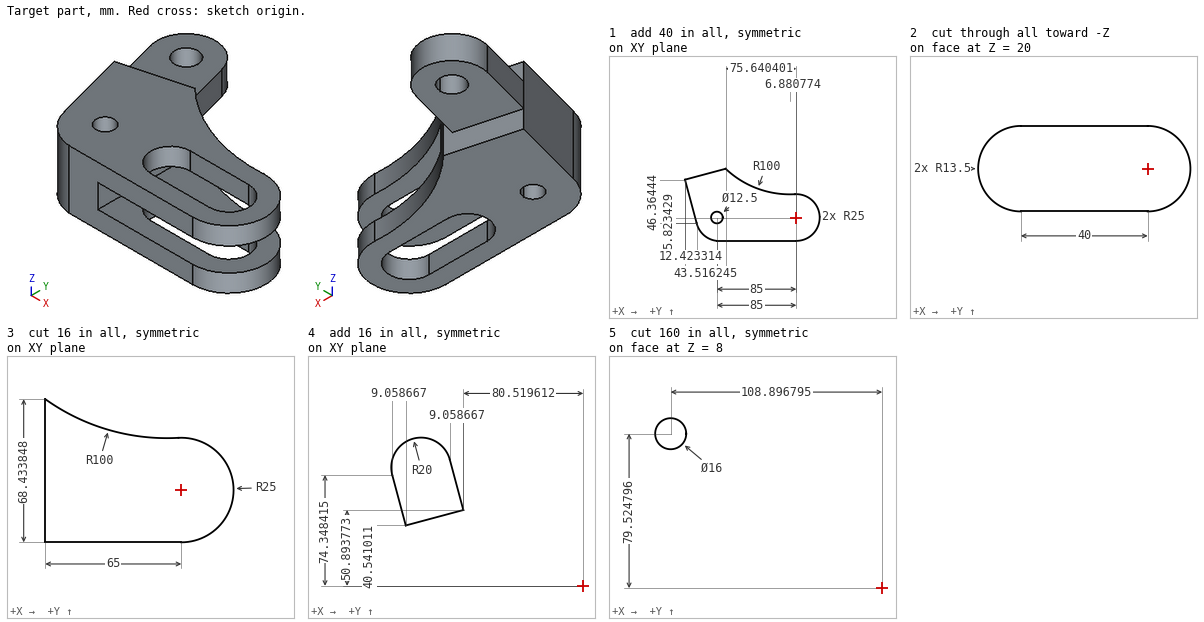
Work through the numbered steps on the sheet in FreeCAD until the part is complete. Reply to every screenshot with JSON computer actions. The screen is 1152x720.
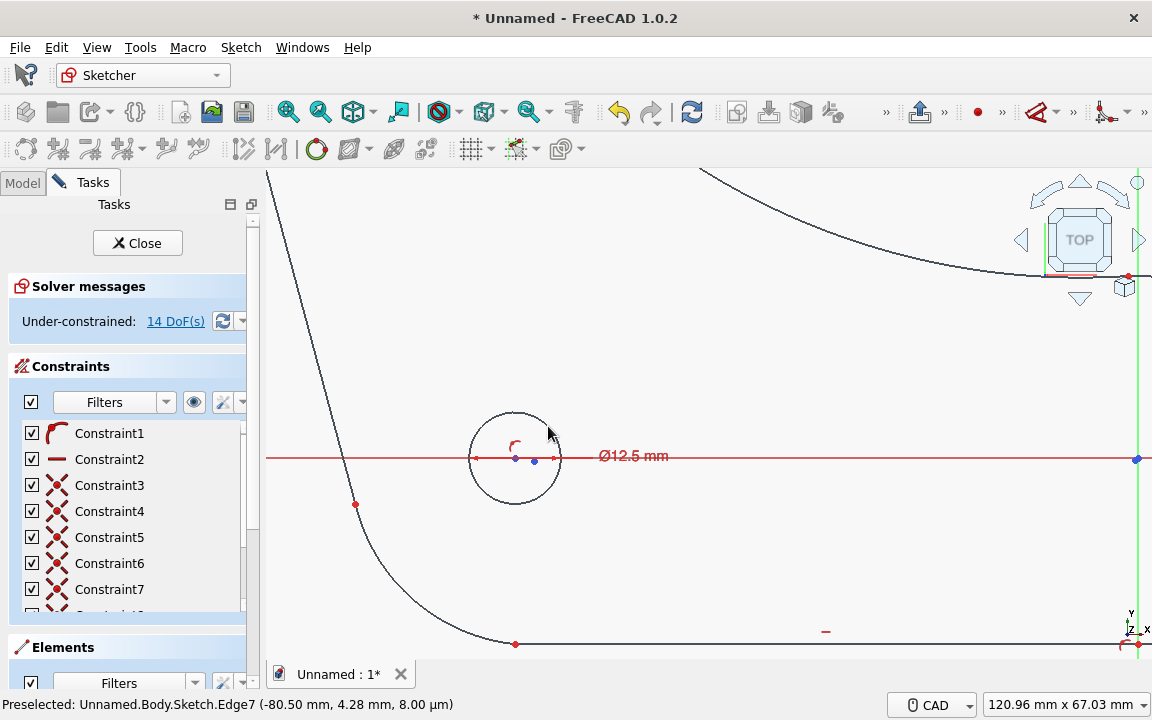
{"action": "scroll", "coordinate": [516, 458], "scroll_direction": "down", "scroll_amount": 4}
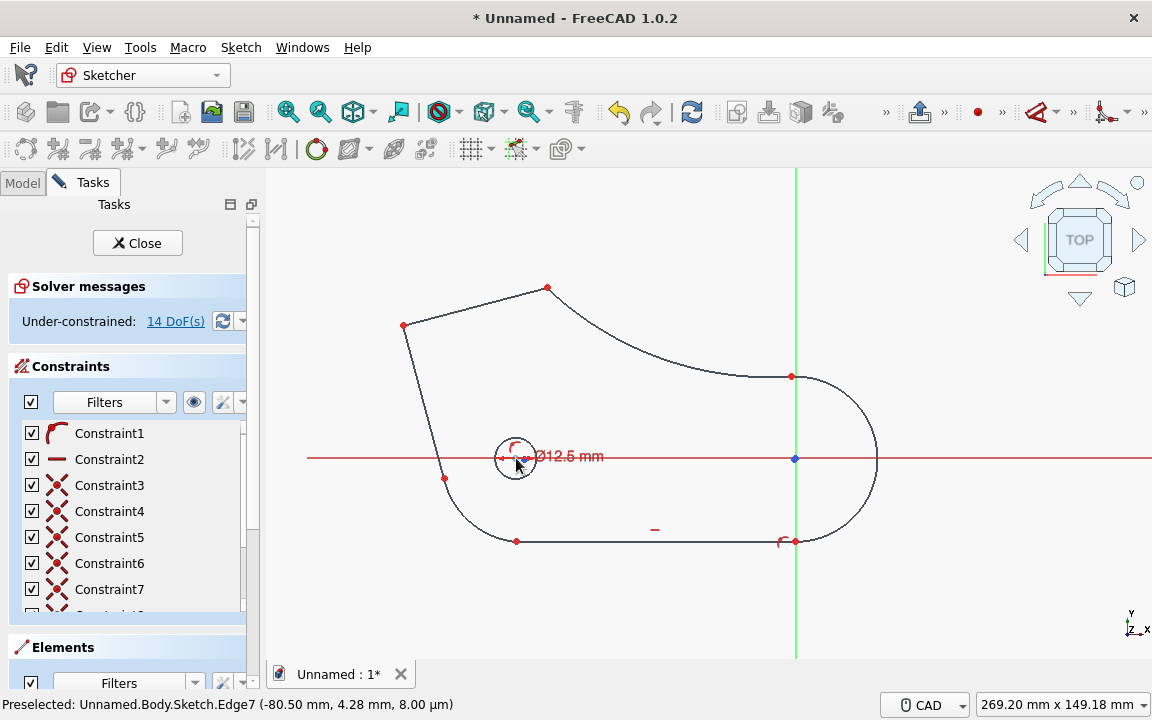
{"action": "left_click", "coordinate": [600, 542]}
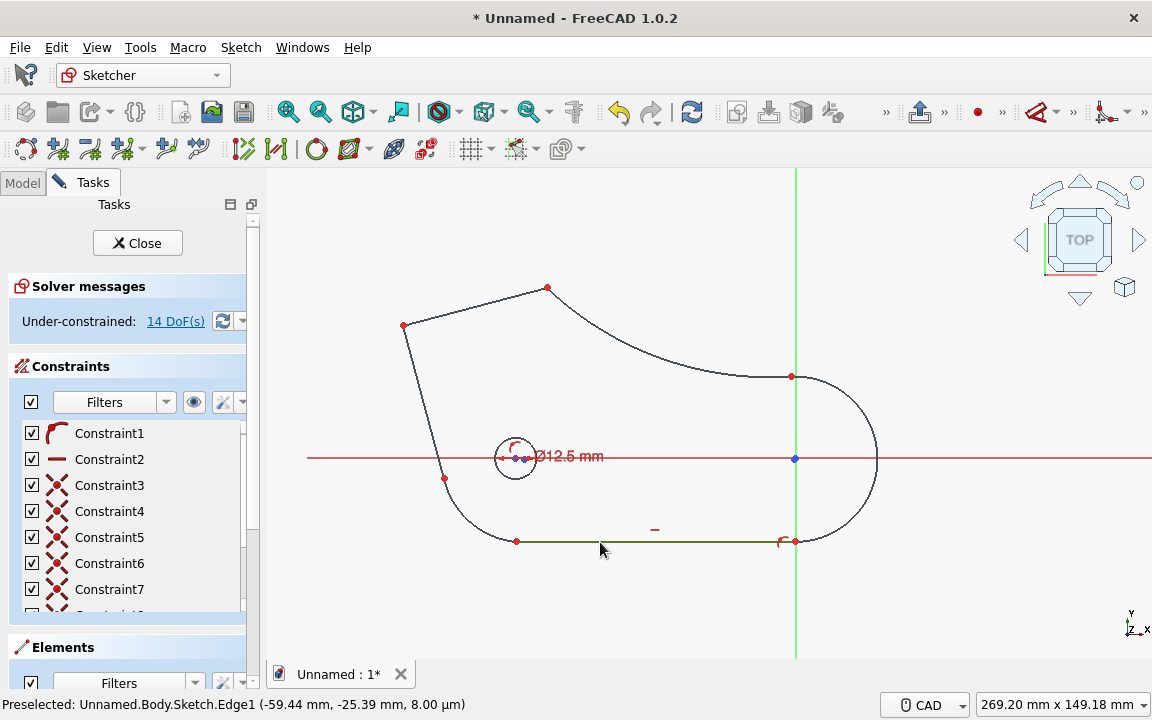
{"action": "left_click", "coordinate": [863, 507]}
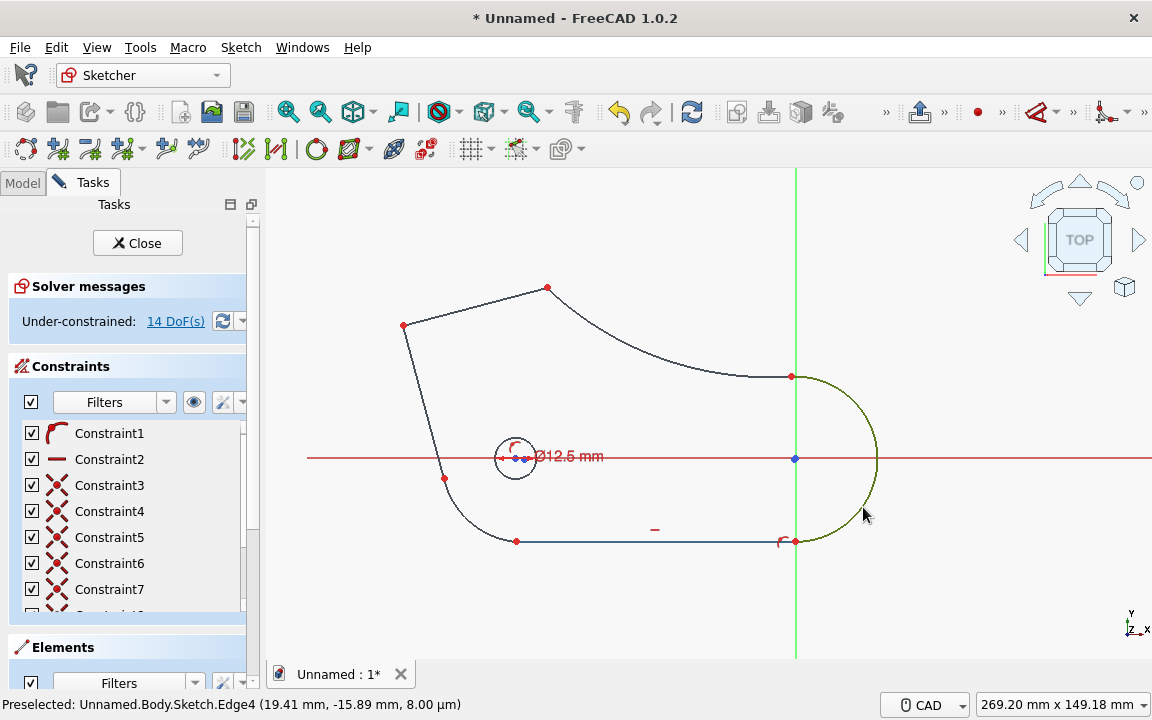
{"action": "key", "text": "t"}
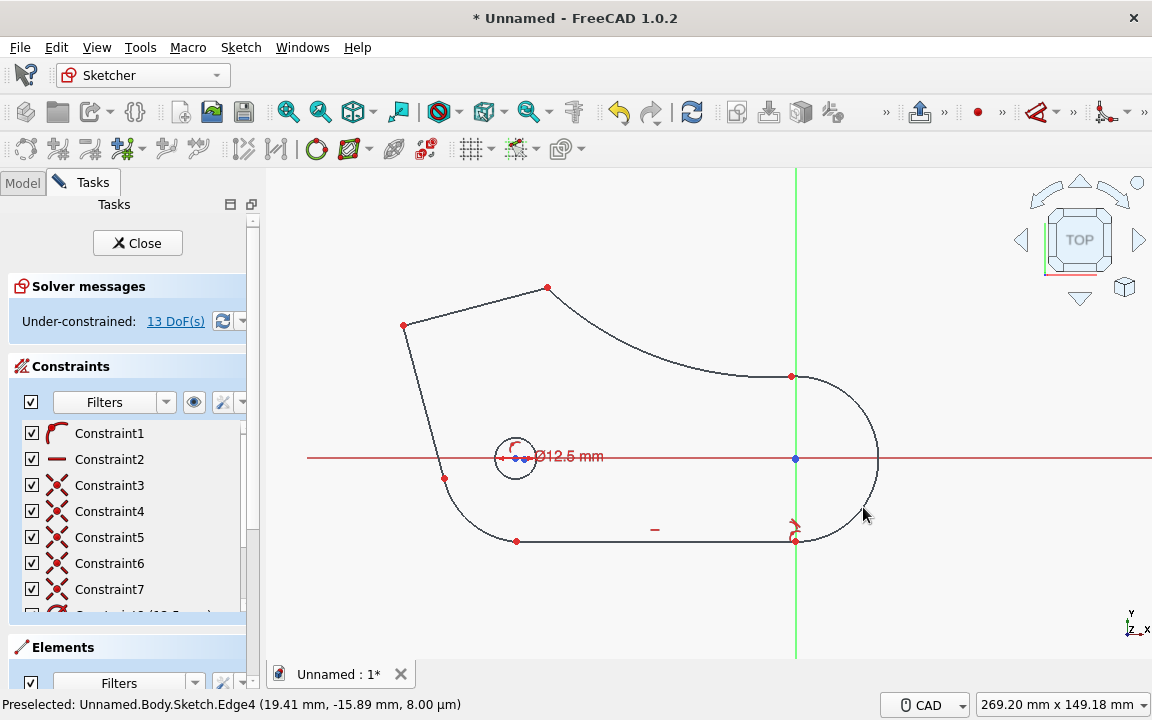
{"action": "left_click", "coordinate": [863, 507]}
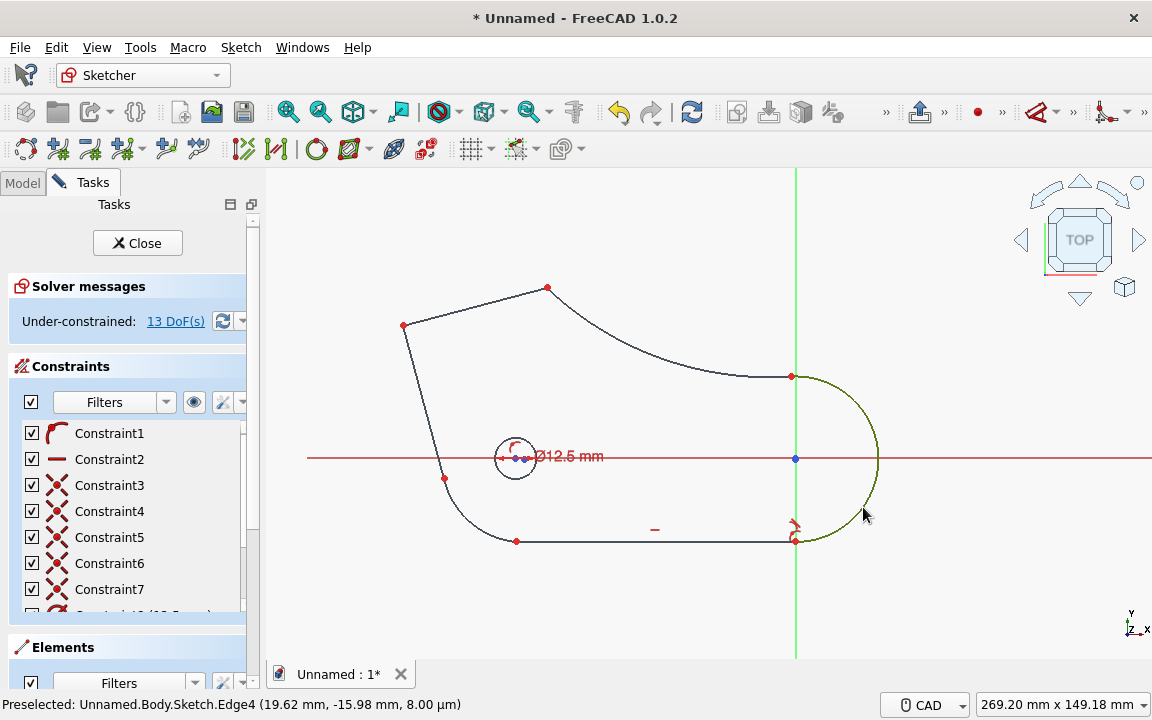
{"action": "left_click", "coordinate": [611, 336]}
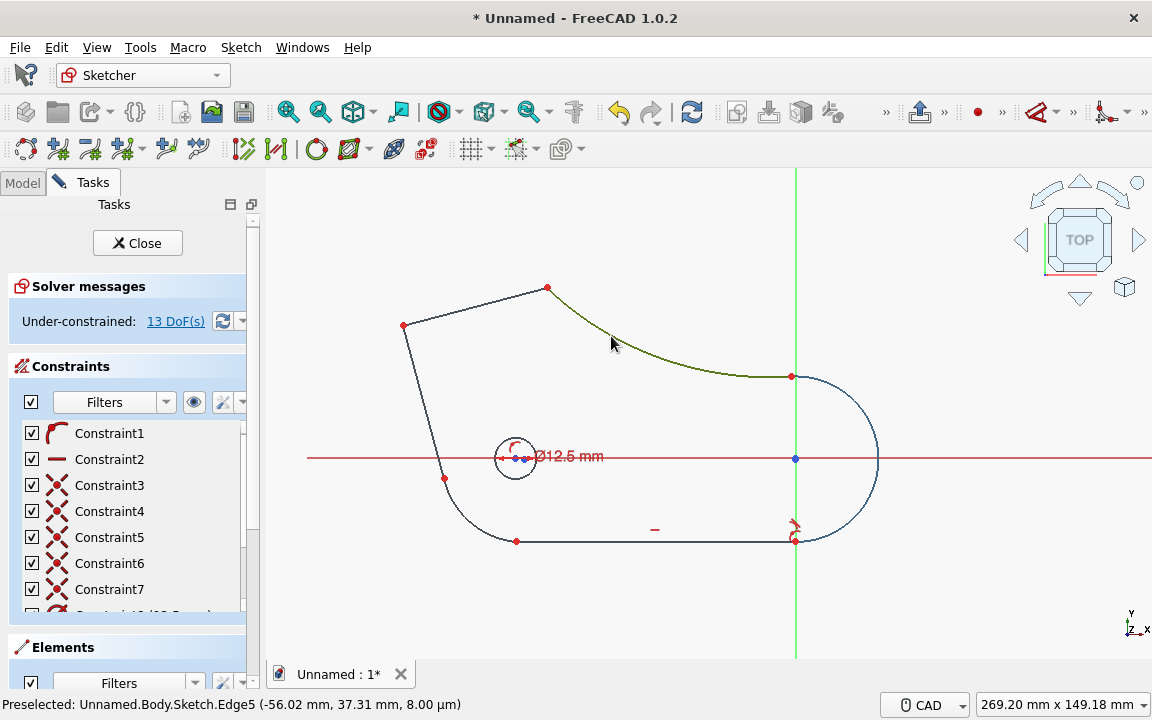
{"action": "key", "text": "t"}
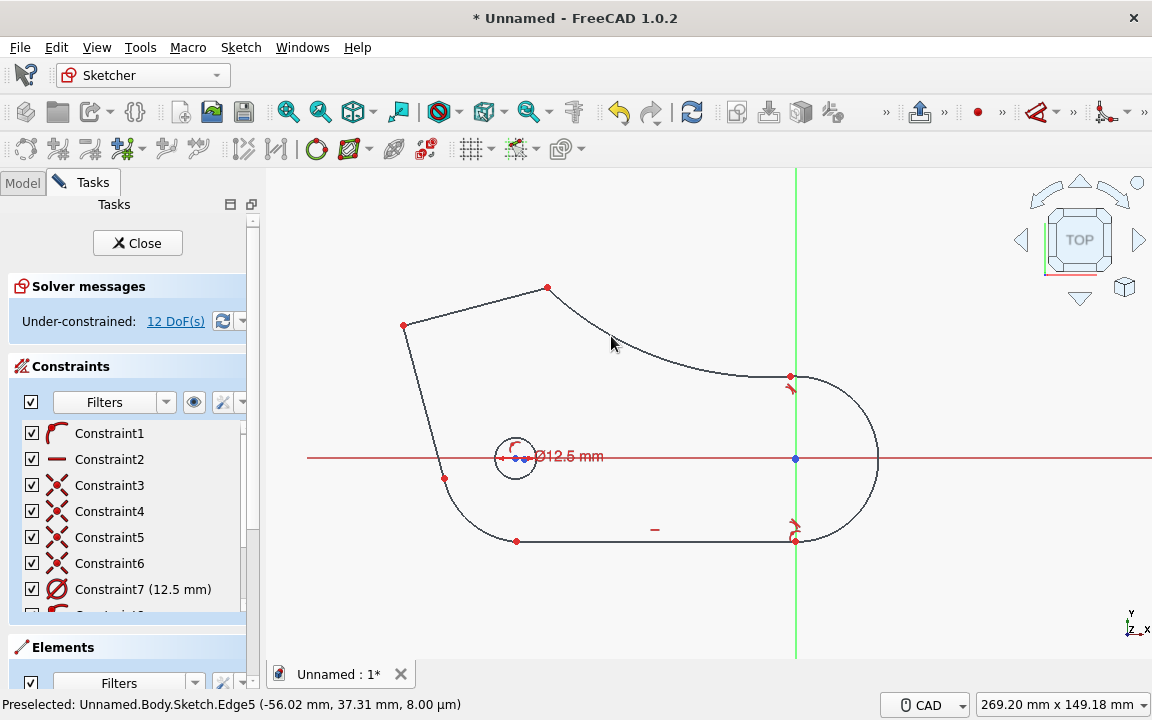
{"action": "left_click", "coordinate": [864, 507]}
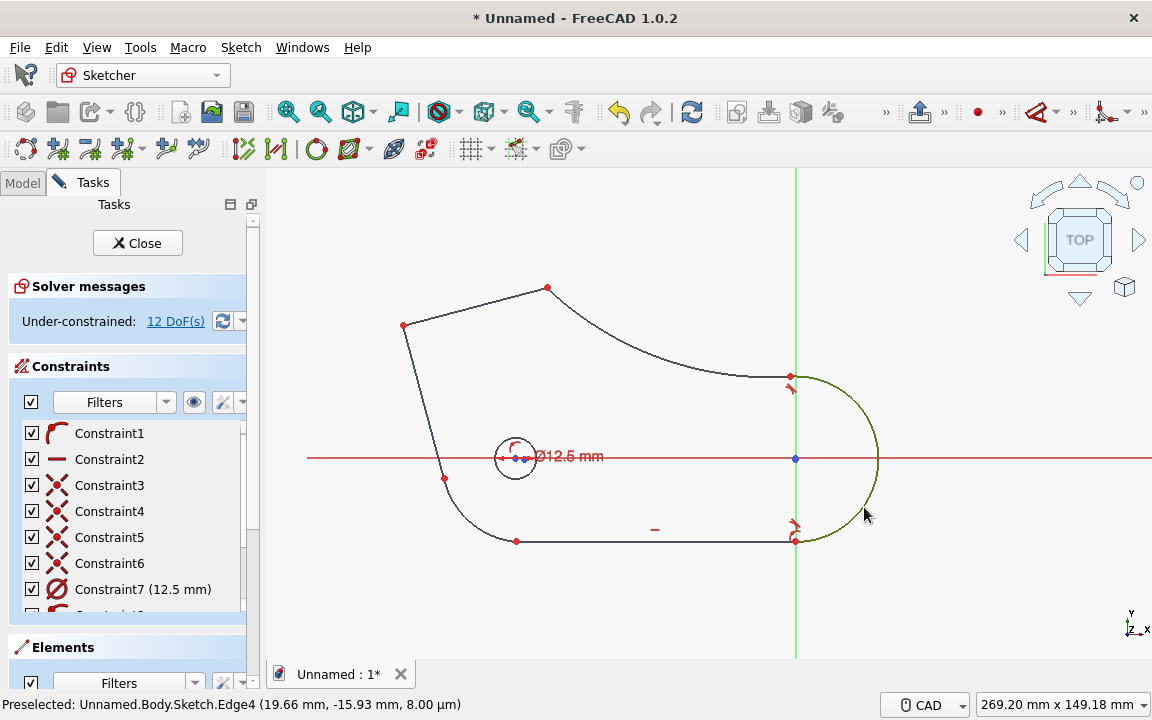
{"action": "left_click", "coordinate": [456, 507]}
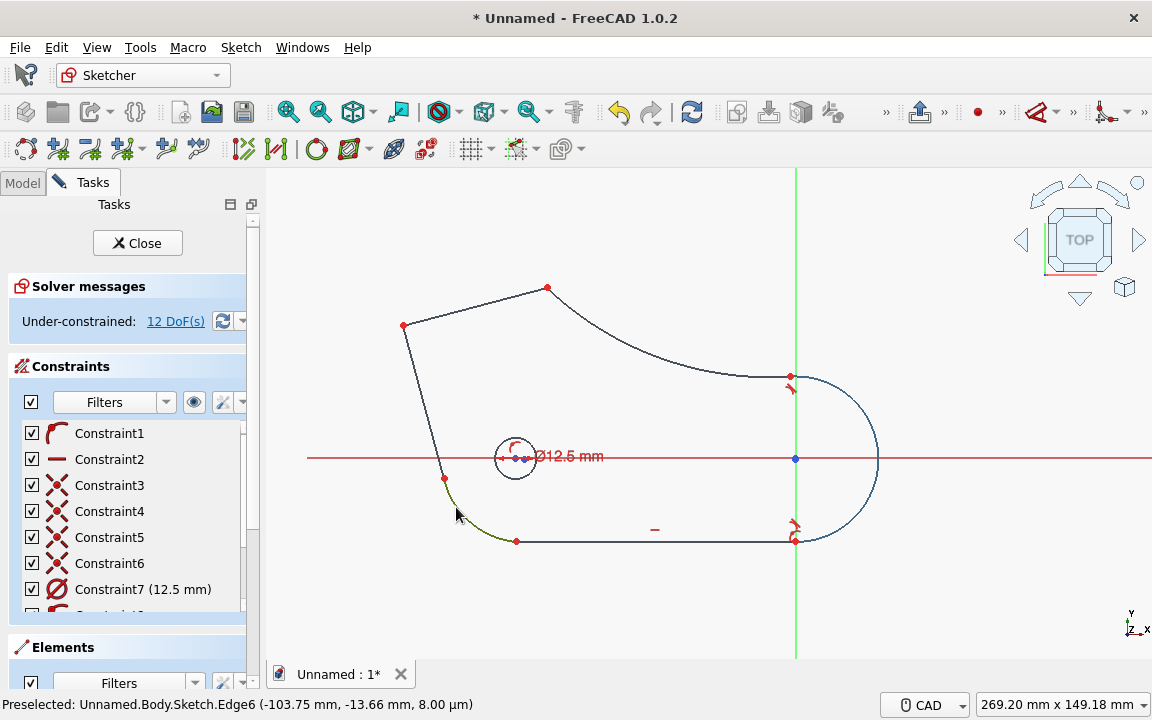
{"action": "key", "text": "e"}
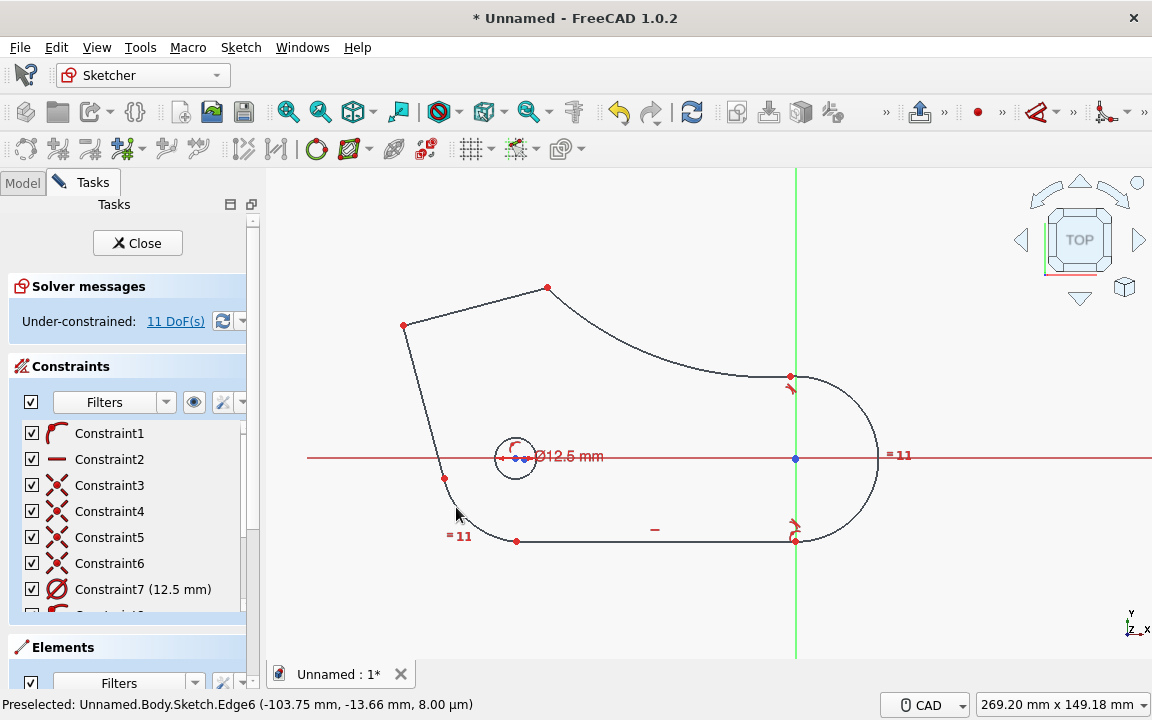
{"action": "left_click", "coordinate": [796, 459]}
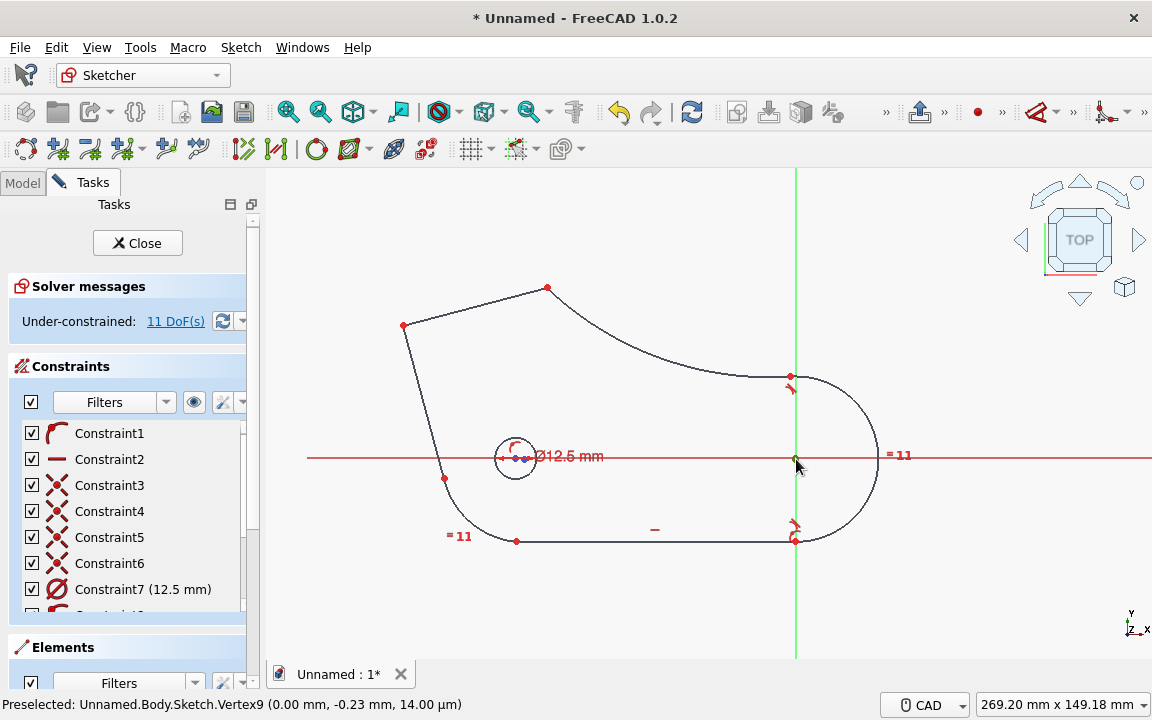
{"action": "left_click", "coordinate": [343, 458]}